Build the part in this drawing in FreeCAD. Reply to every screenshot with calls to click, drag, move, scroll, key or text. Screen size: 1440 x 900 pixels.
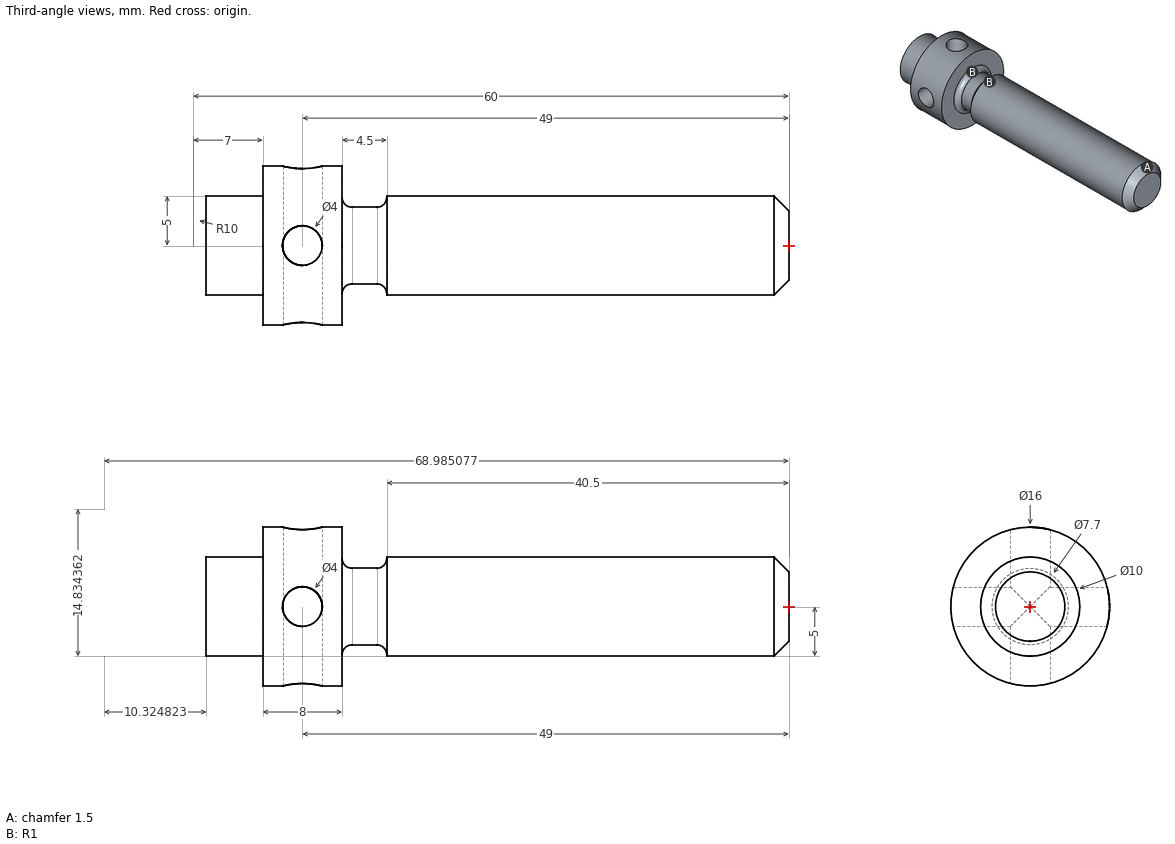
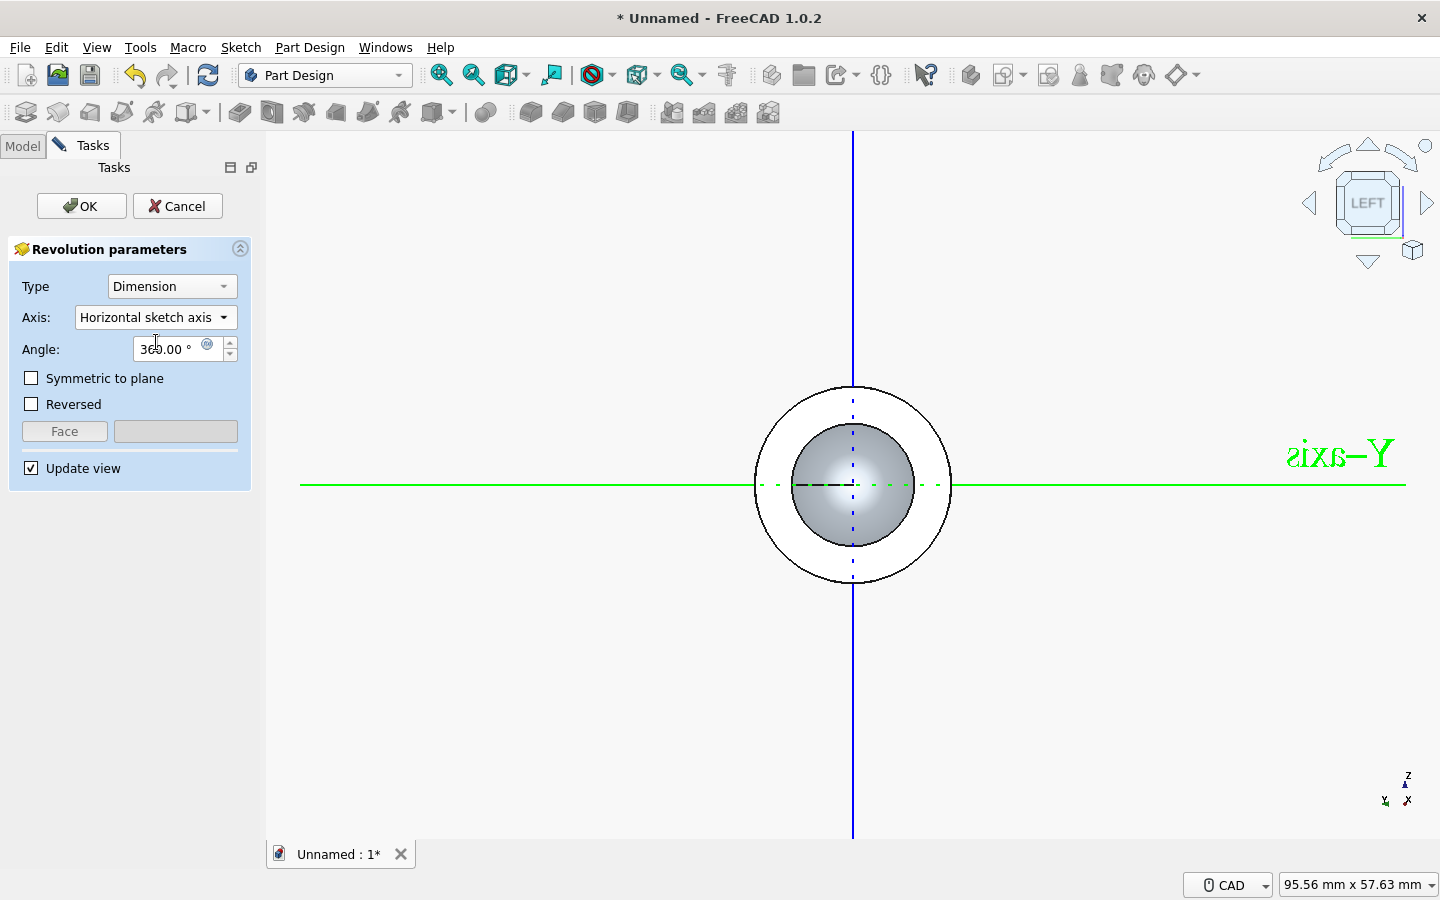
click(82, 206)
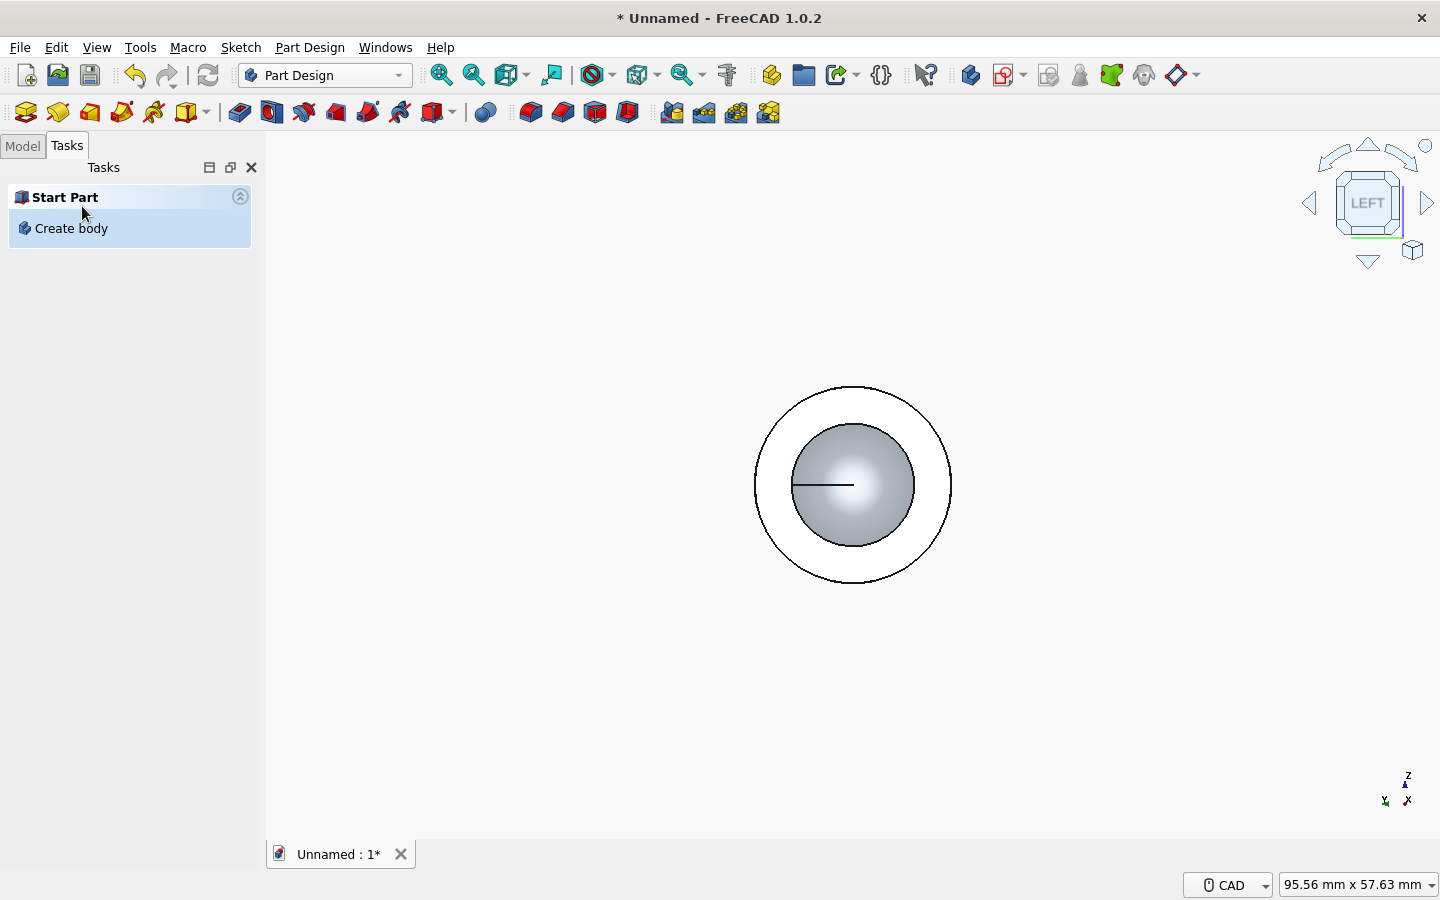
key(v)
key(f)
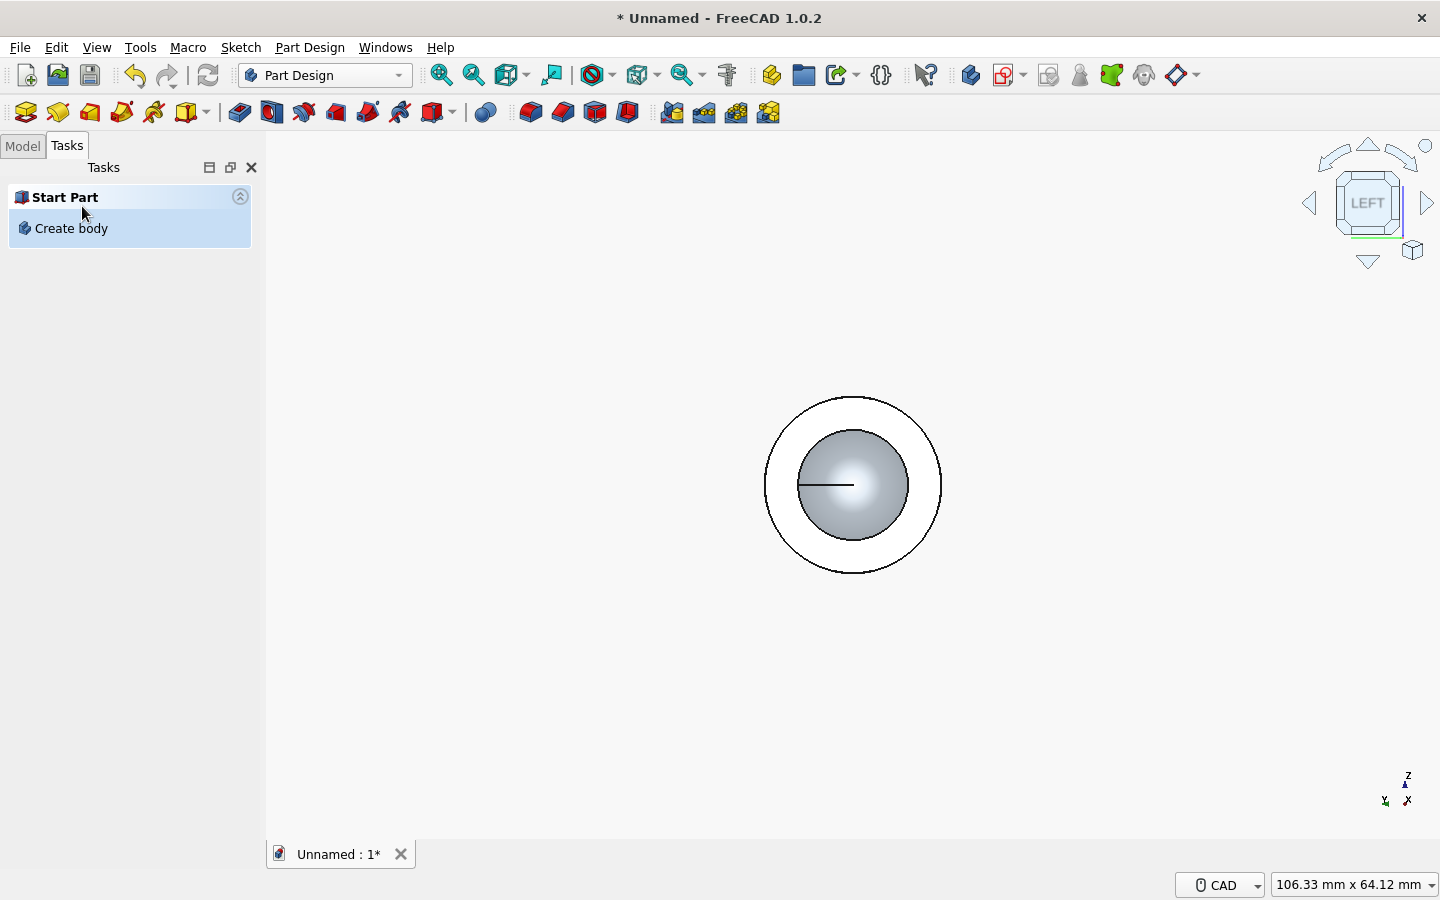
key(0)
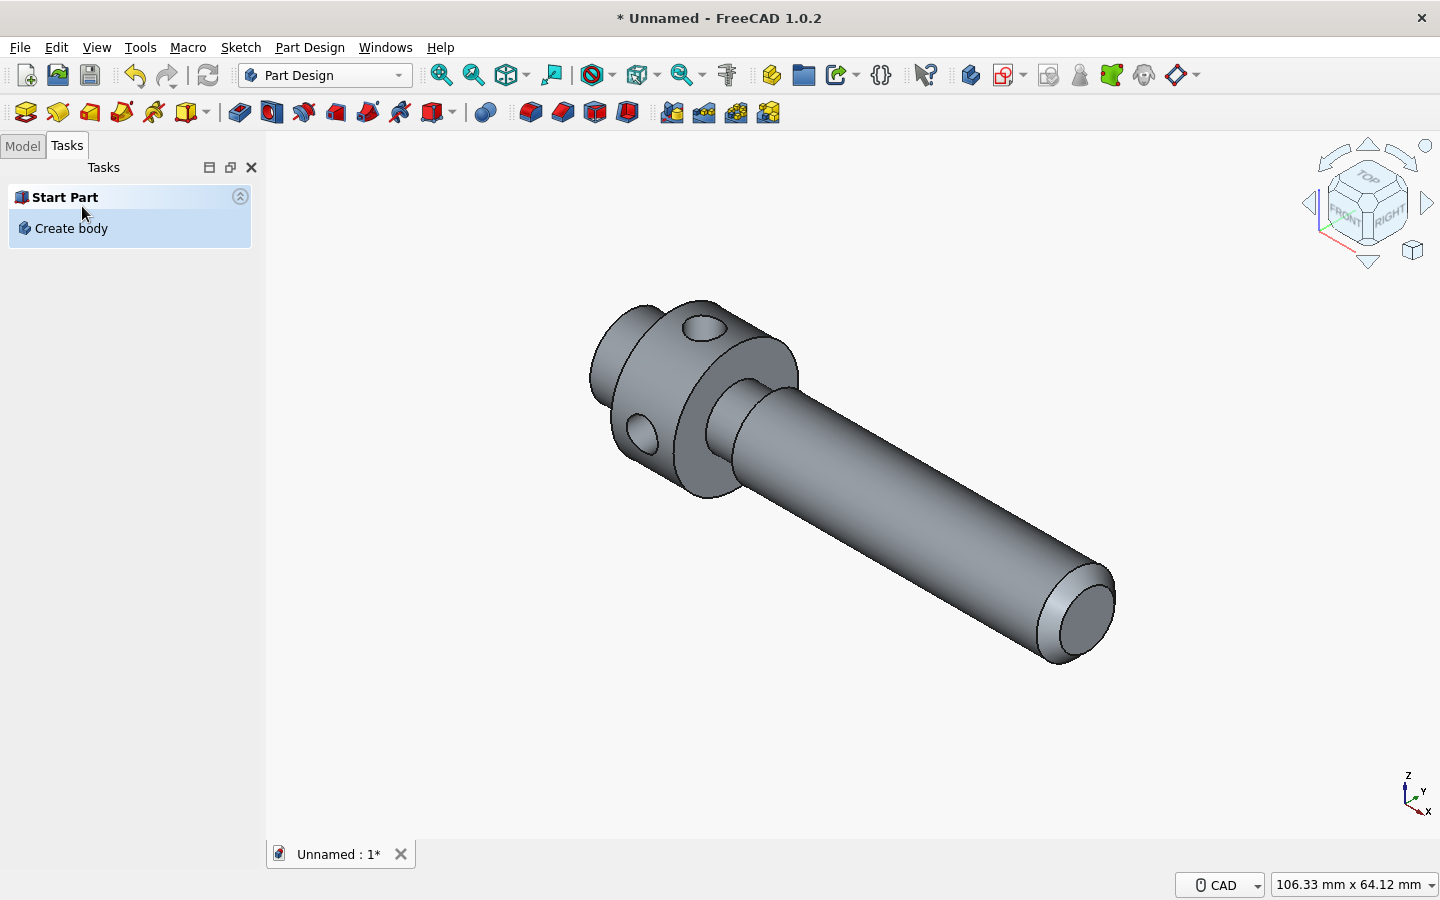
key(2)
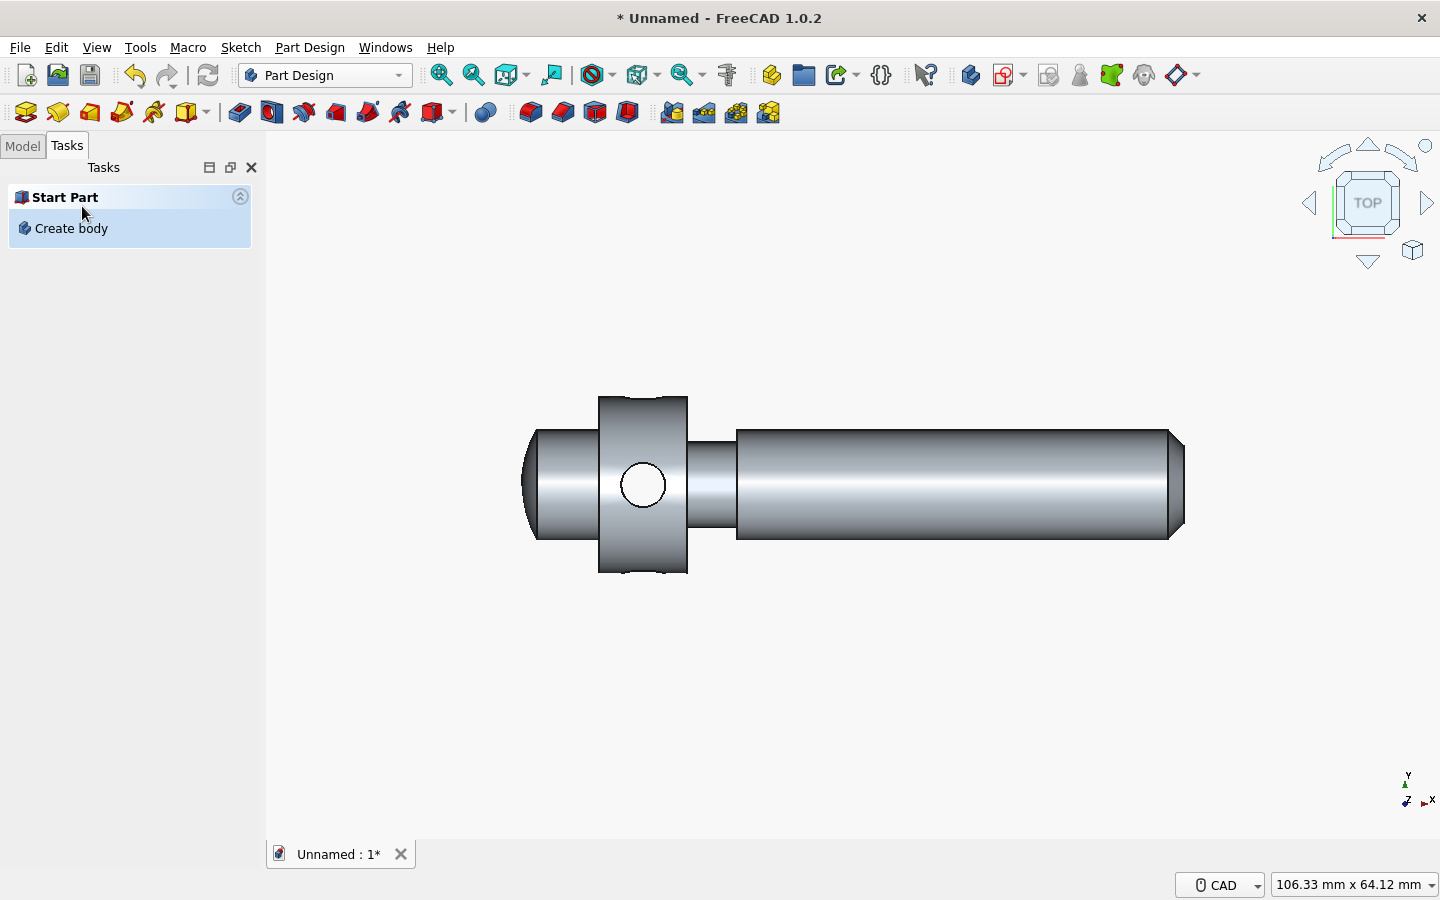
key(1)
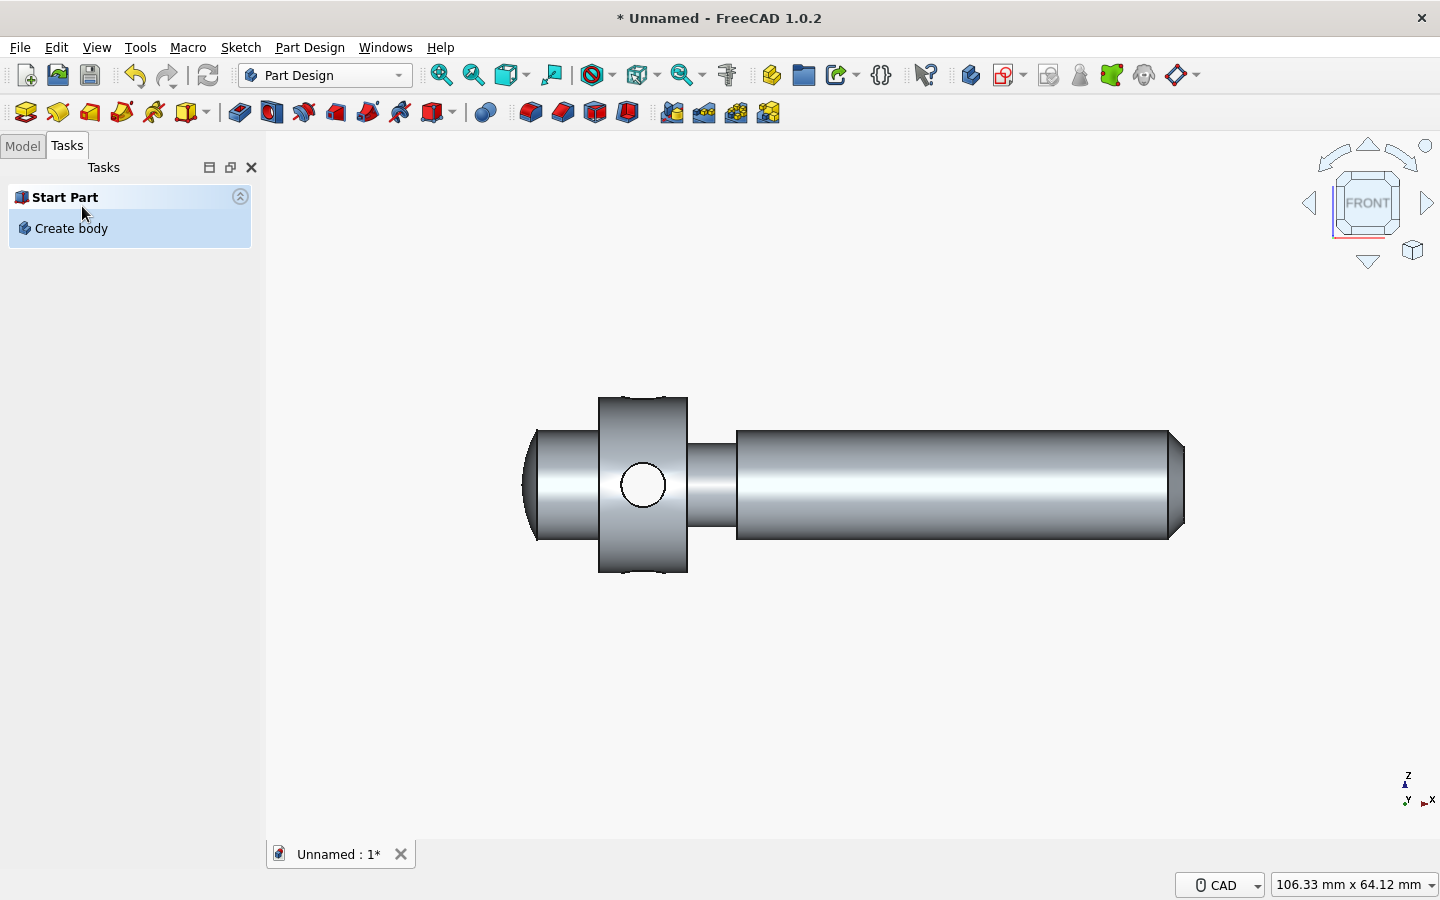
key(3)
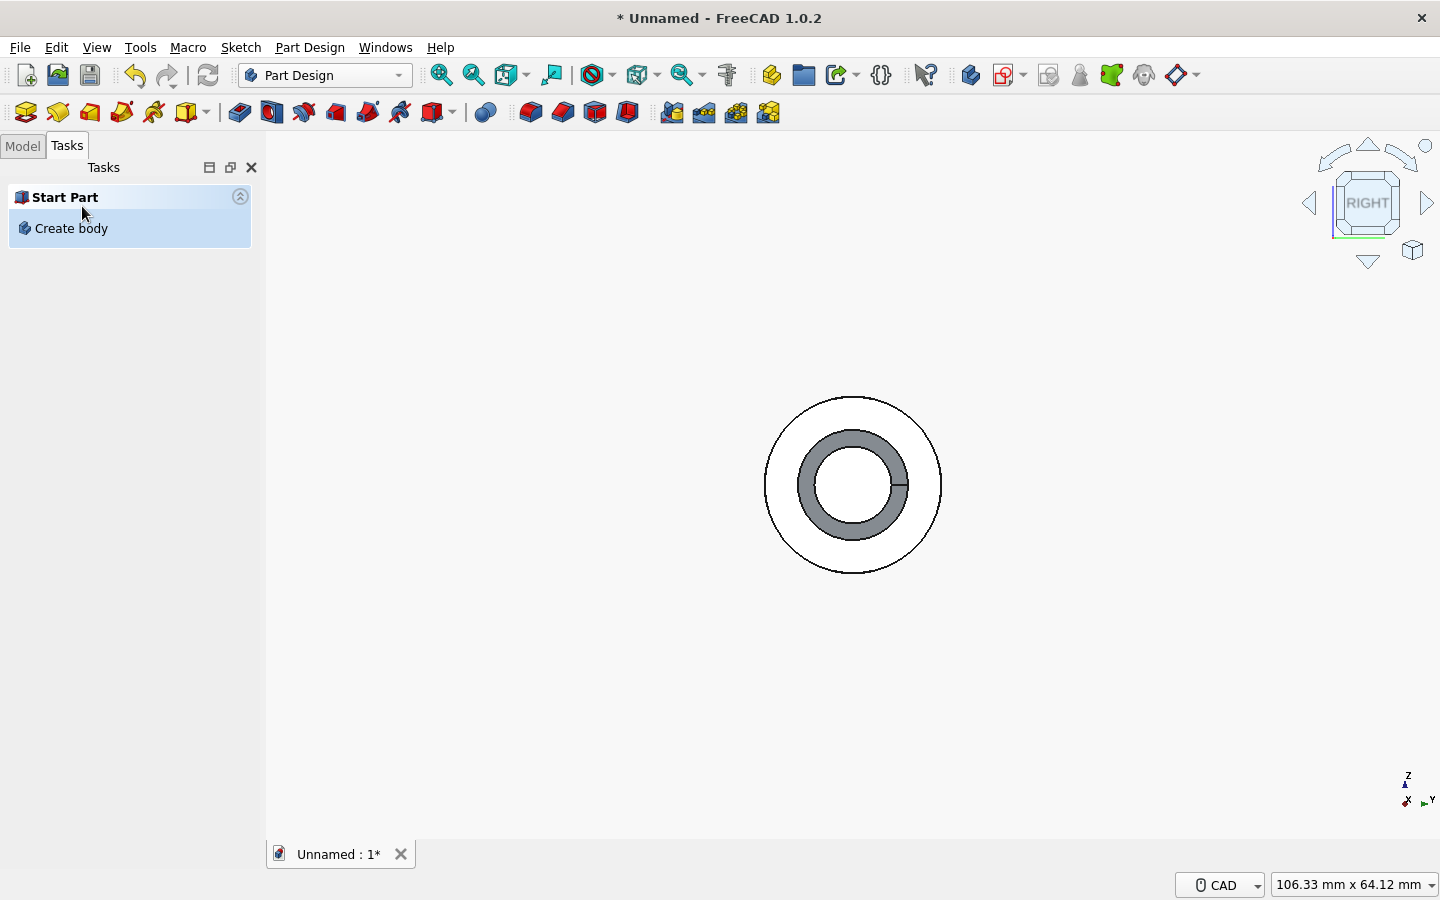
key(v)
key(f)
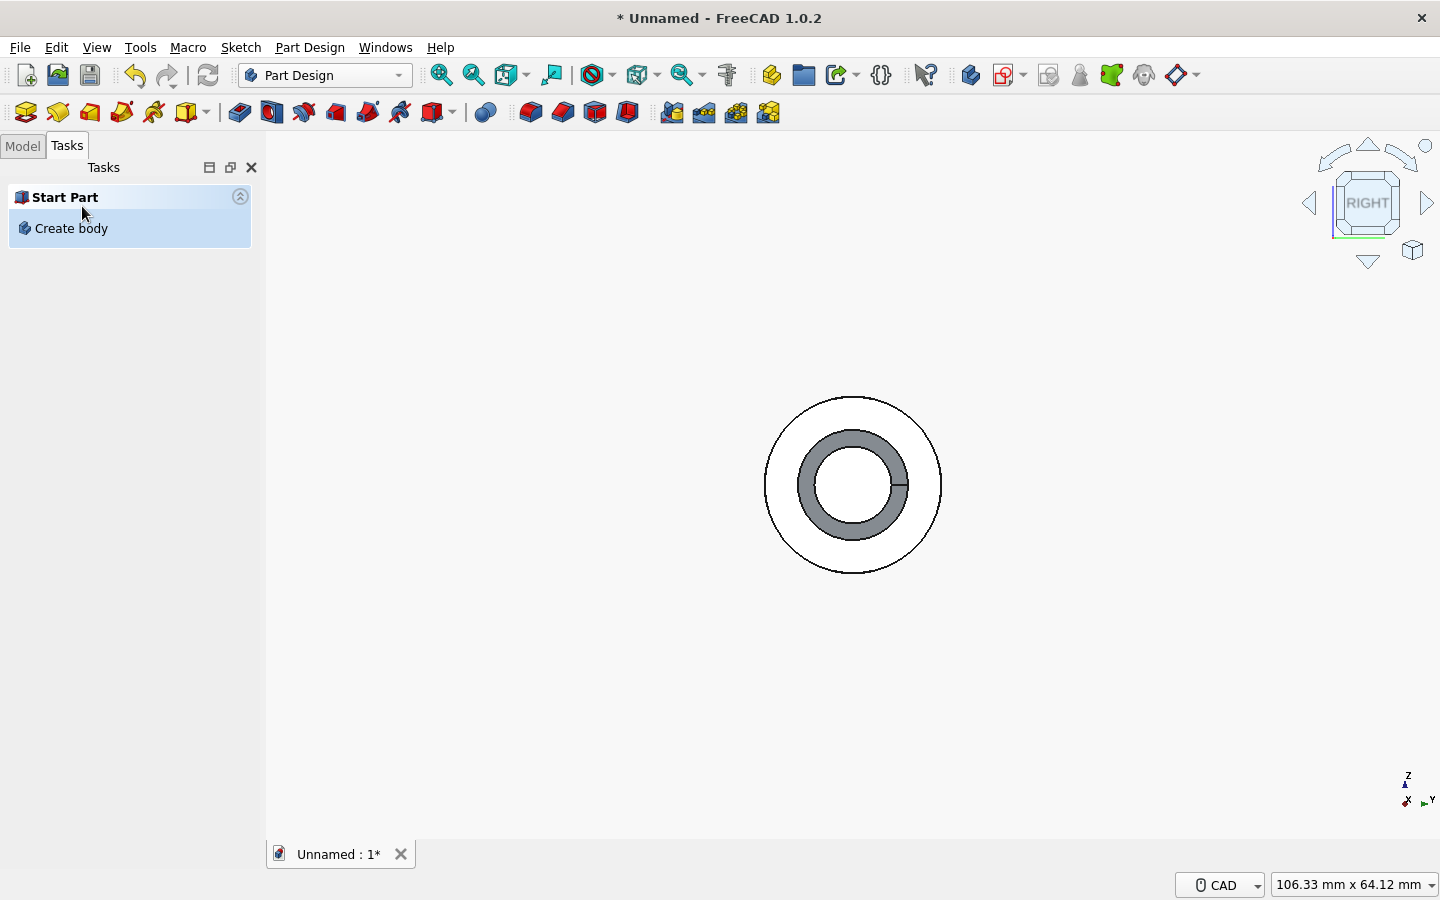
key(5)